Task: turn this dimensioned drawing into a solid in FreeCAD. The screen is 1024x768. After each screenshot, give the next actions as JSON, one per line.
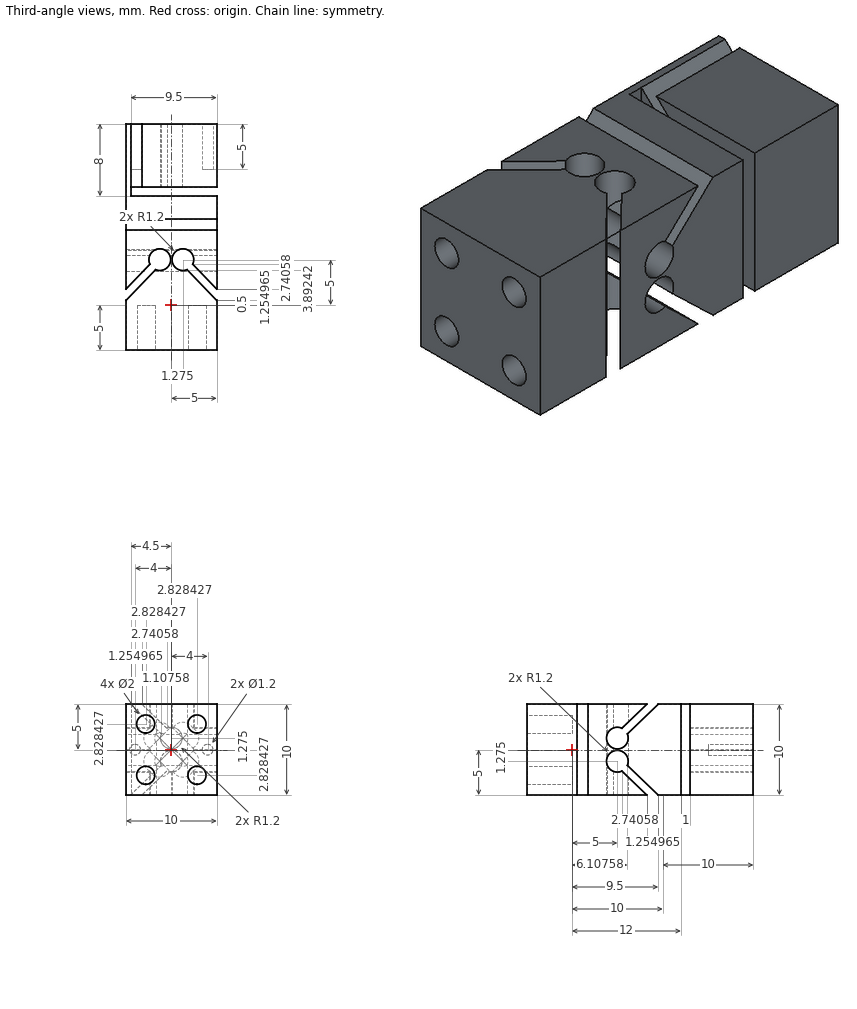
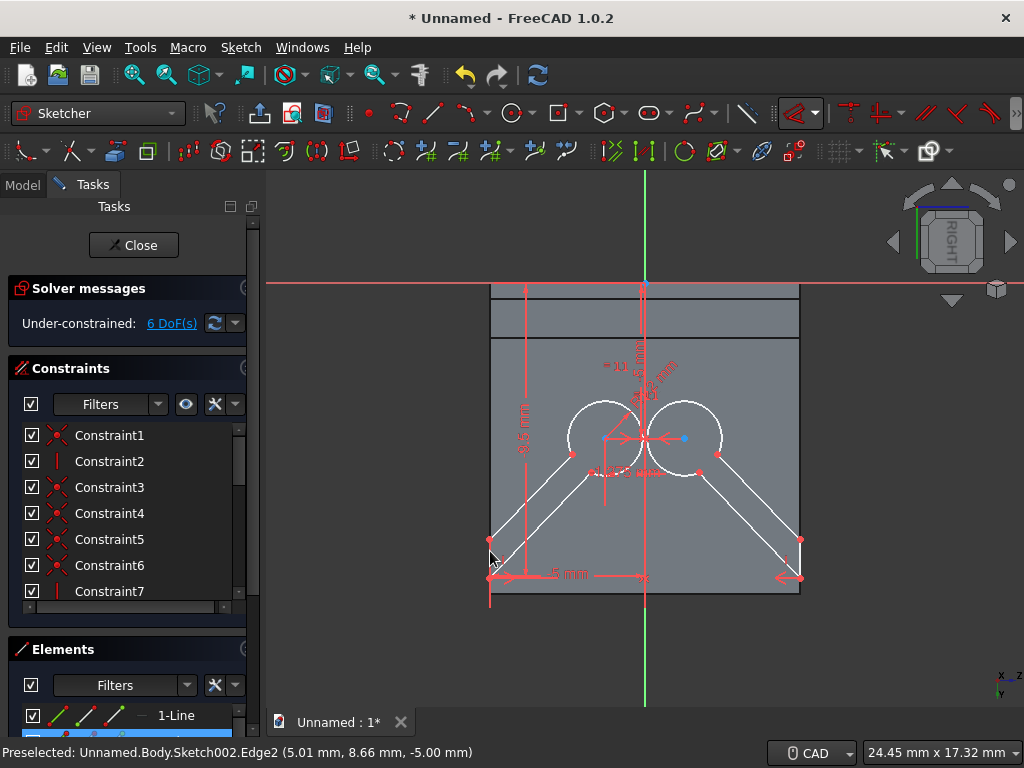
{"action": "left_click", "coordinate": [818, 114]}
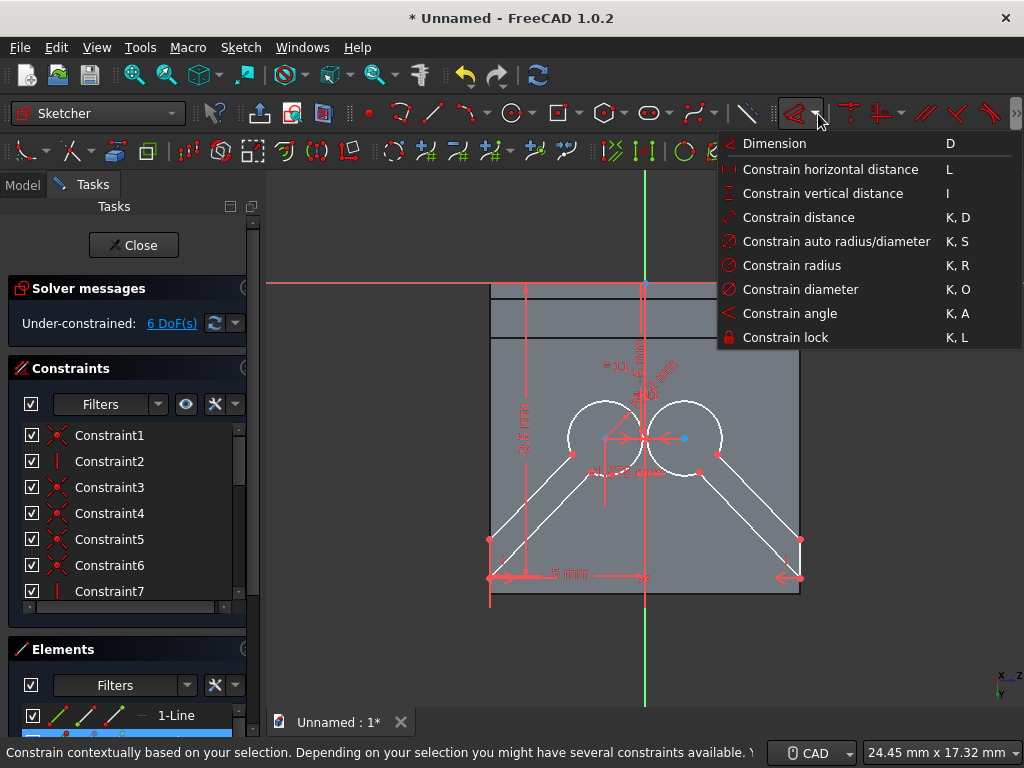
{"action": "left_click", "coordinate": [870, 193]}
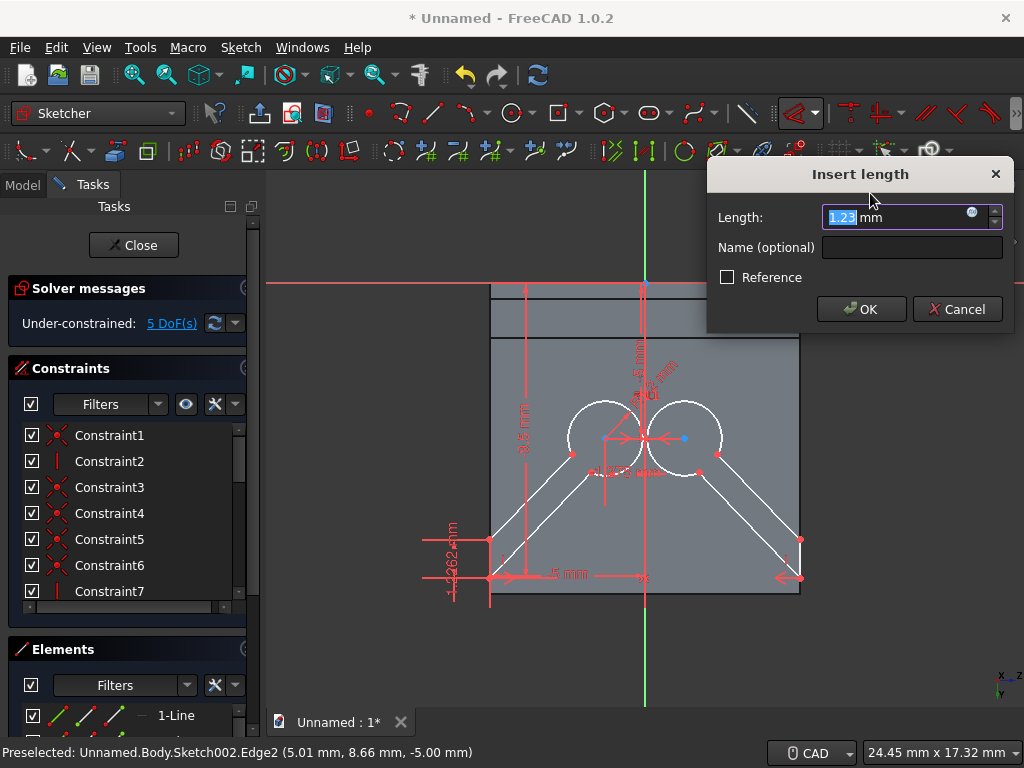
{"action": "type", "text": "1.254965"}
{"action": "key", "text": "Return"}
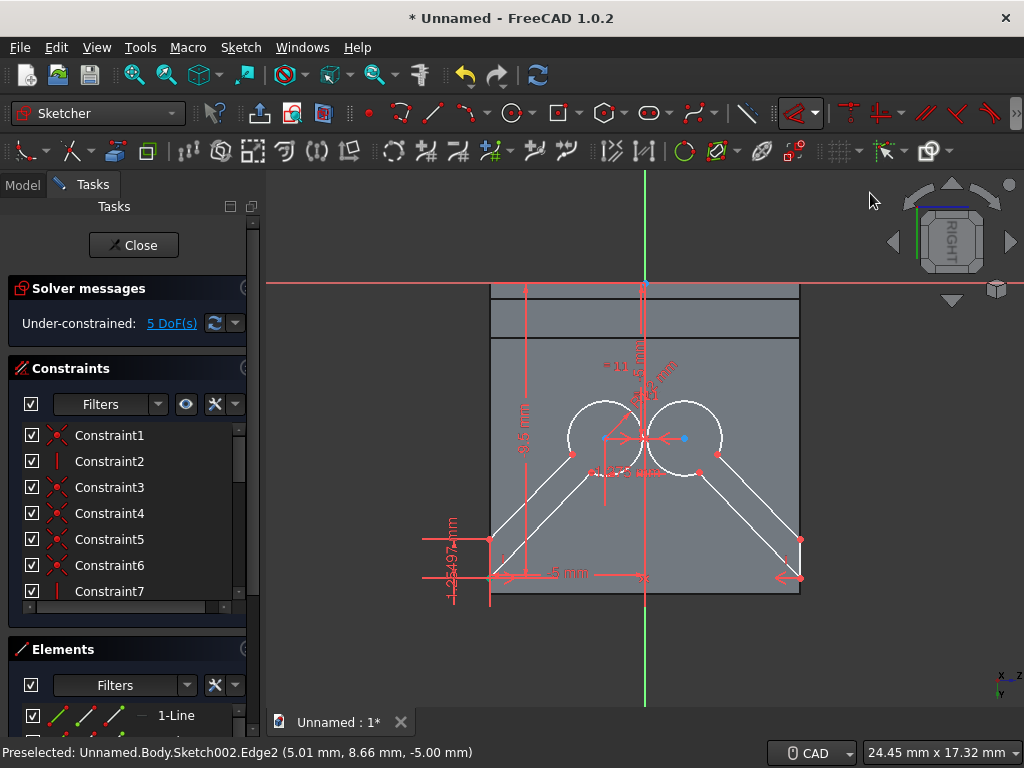
{"action": "left_click", "coordinate": [800, 551]}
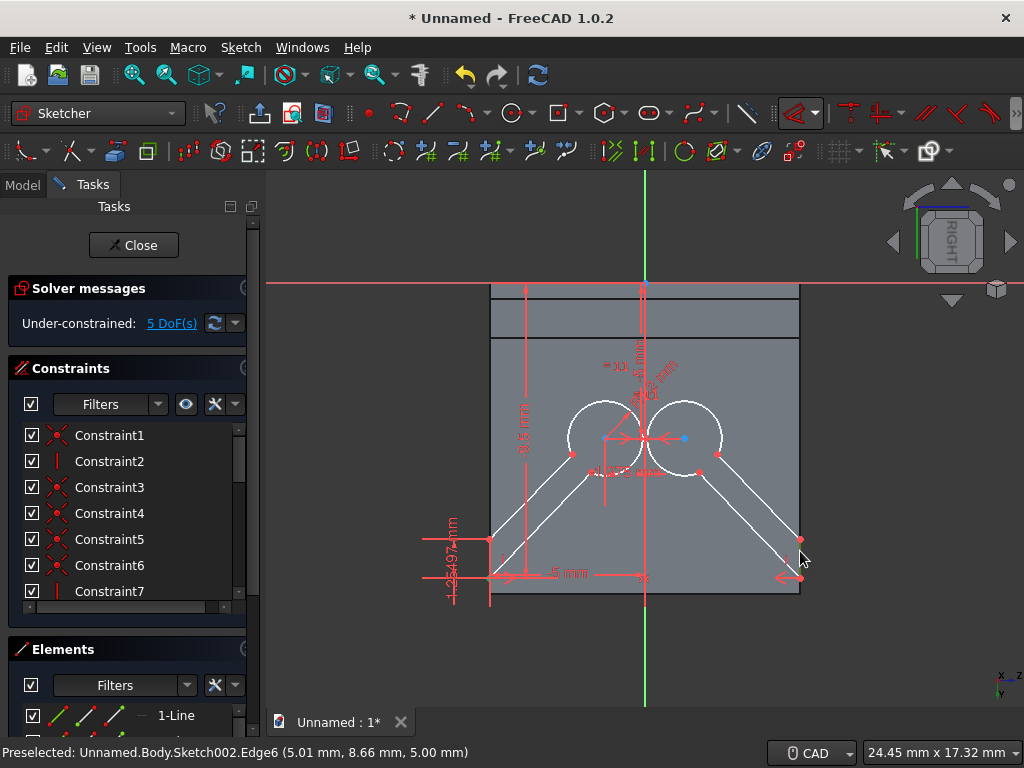
{"action": "left_click", "coordinate": [818, 114]}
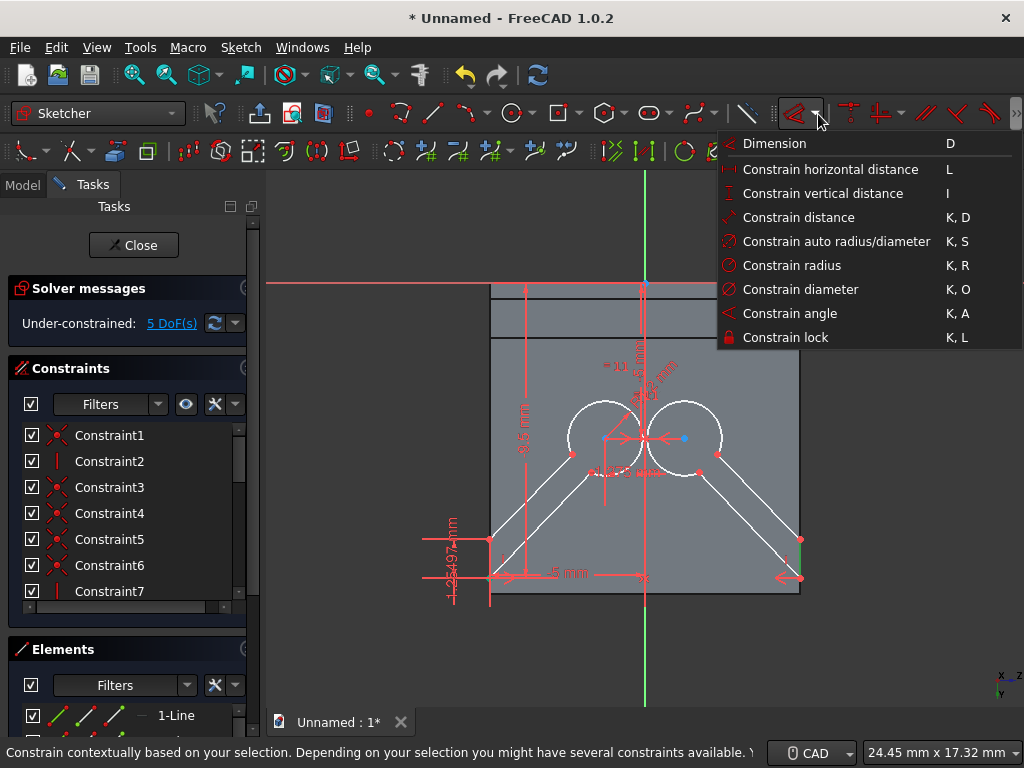
{"action": "left_click", "coordinate": [870, 193]}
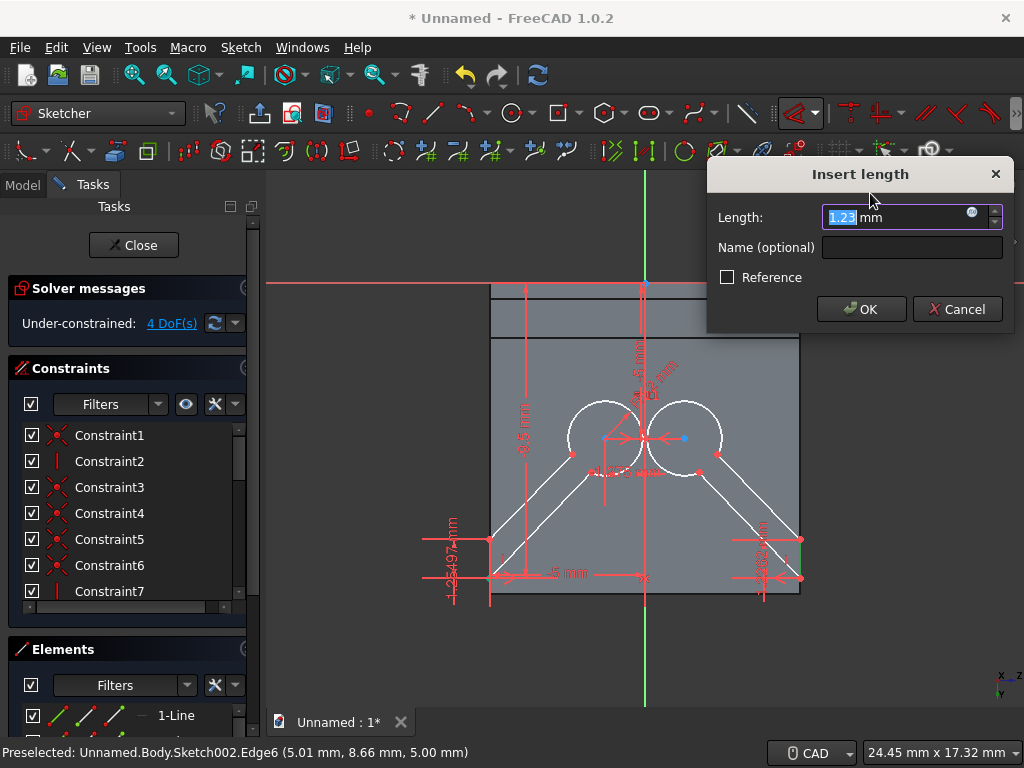
{"action": "type", "text": "1.254965"}
{"action": "key", "text": "Return"}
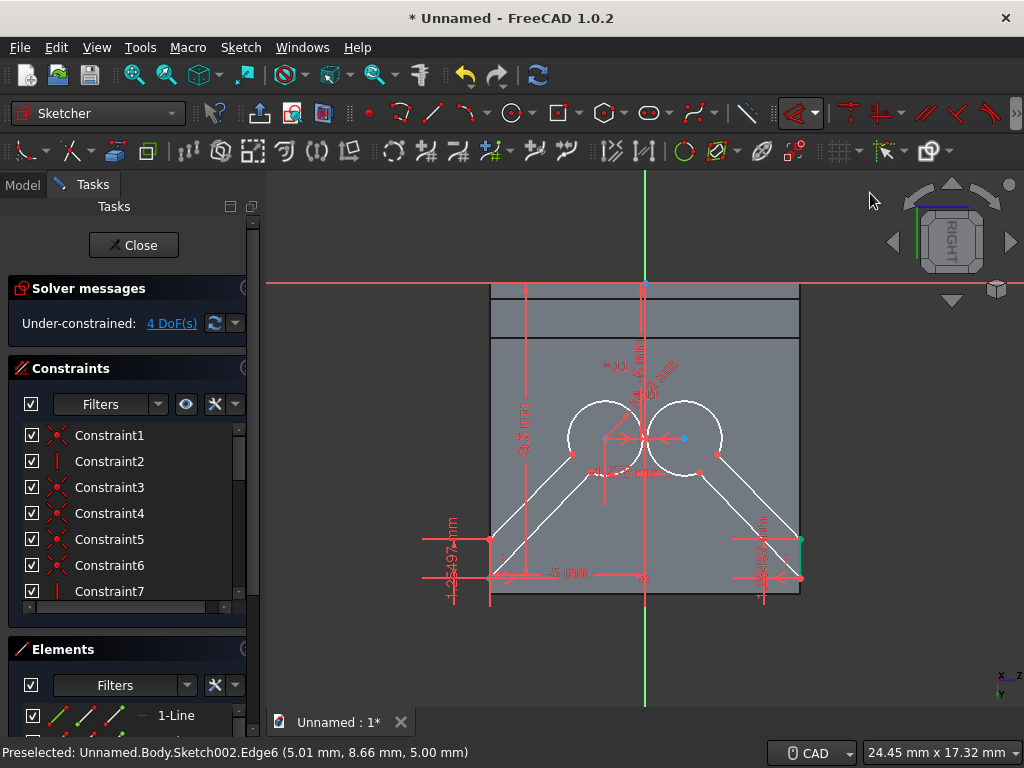
{"action": "left_click", "coordinate": [591, 473]}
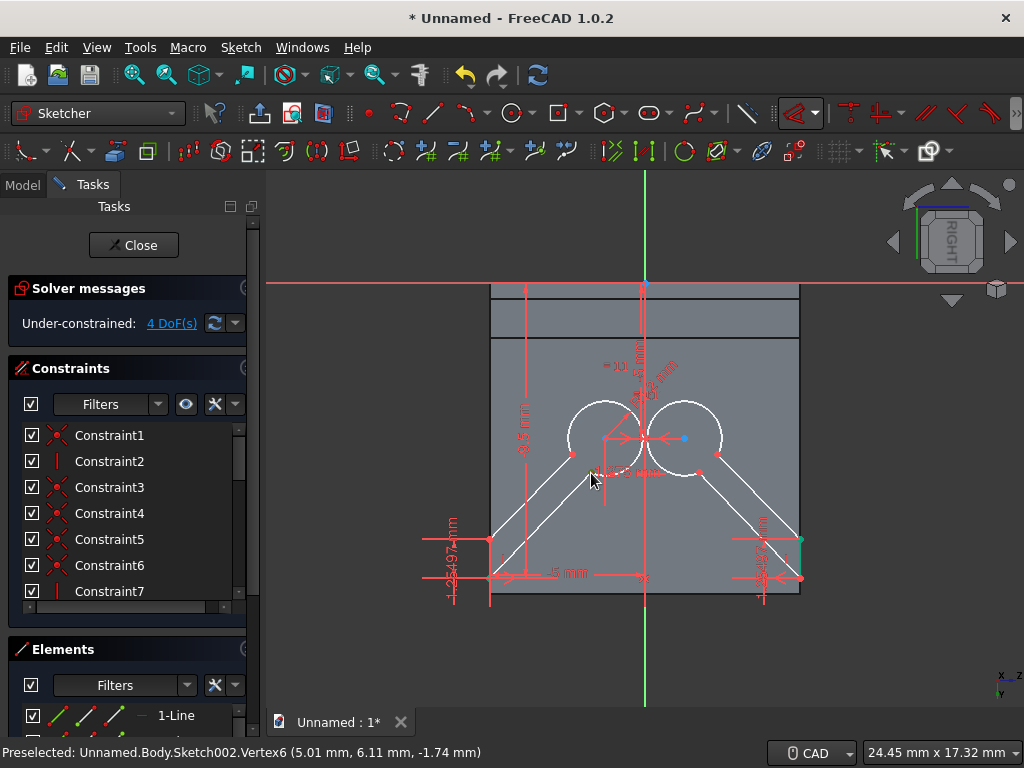
{"action": "left_click", "coordinate": [818, 114]}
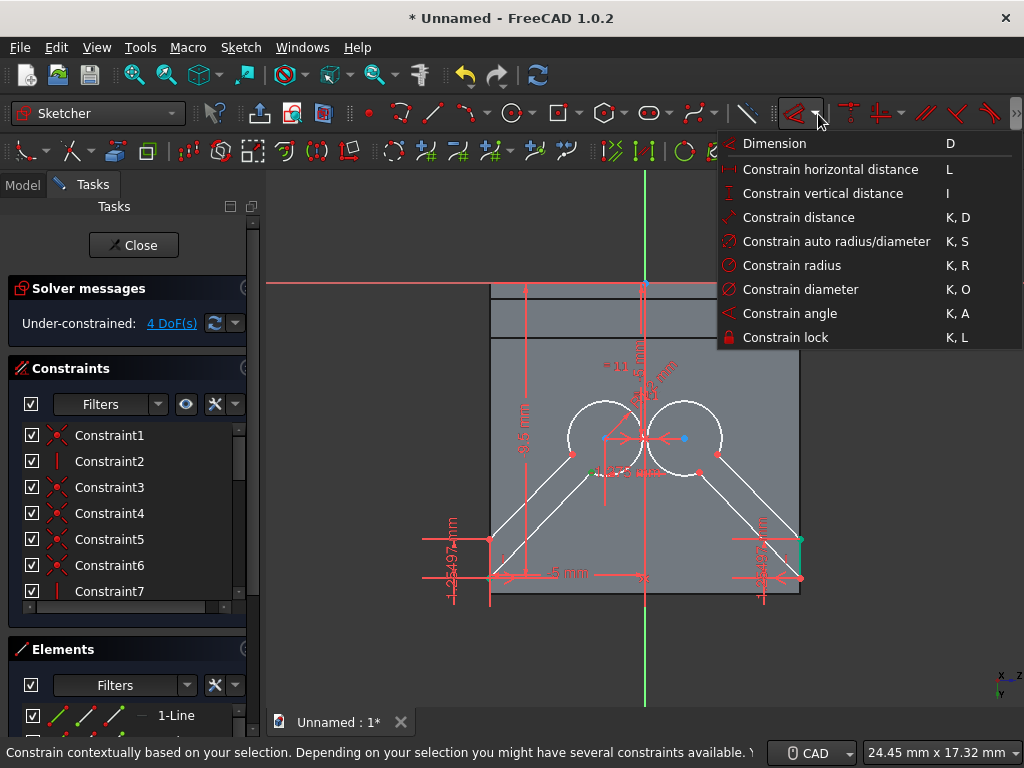
{"action": "left_click", "coordinate": [870, 193]}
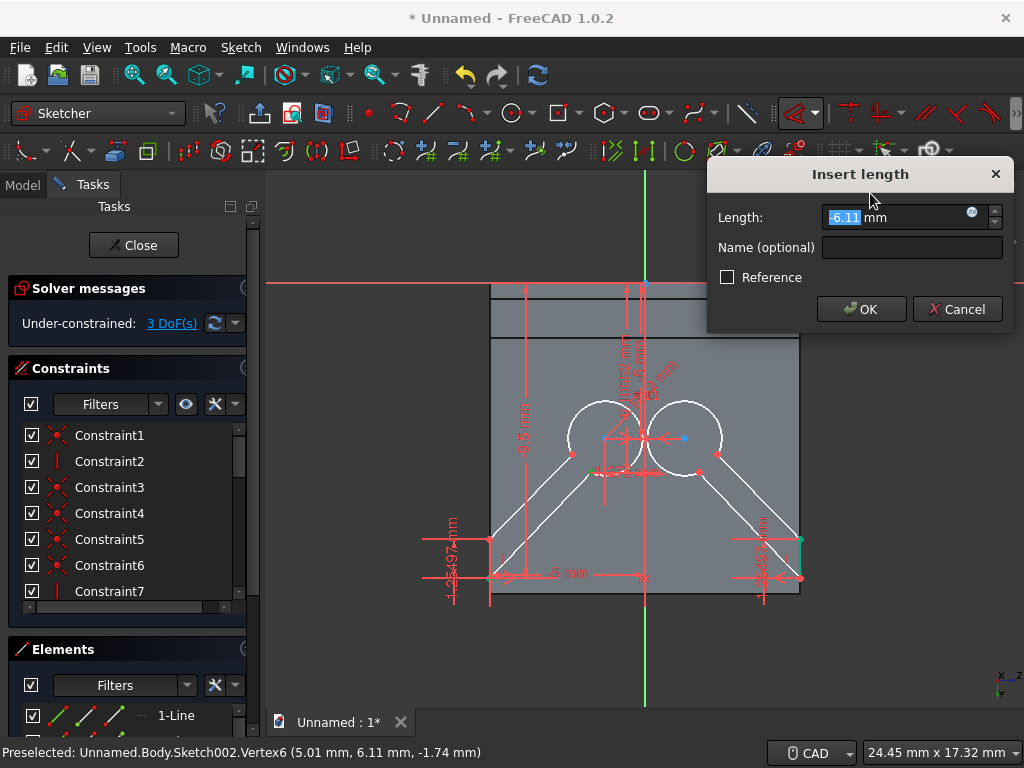
{"action": "type", "text": "-6.10758"}
{"action": "key", "text": "Return"}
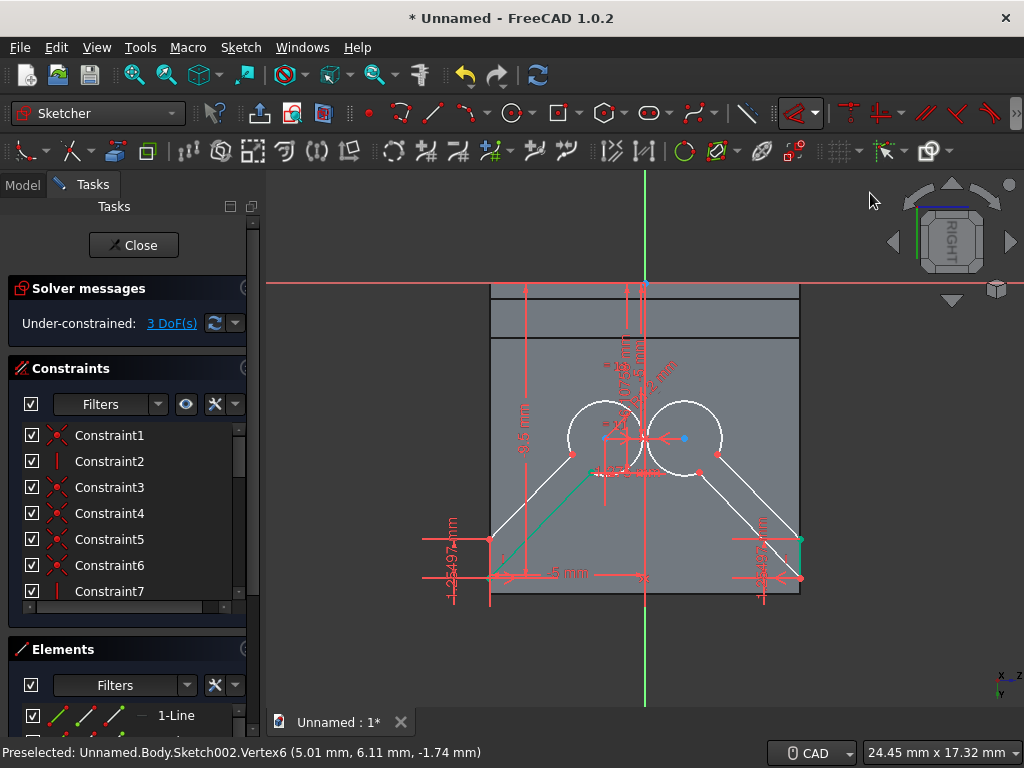
{"action": "left_click", "coordinate": [699, 473]}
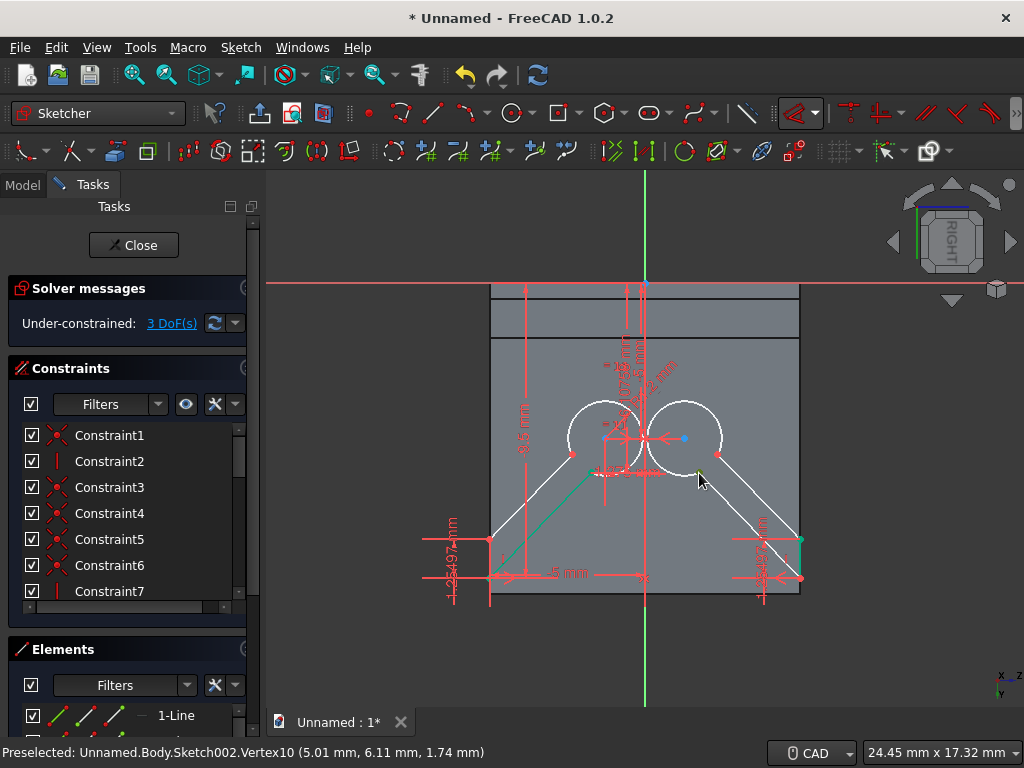
{"action": "key", "text": "i"}